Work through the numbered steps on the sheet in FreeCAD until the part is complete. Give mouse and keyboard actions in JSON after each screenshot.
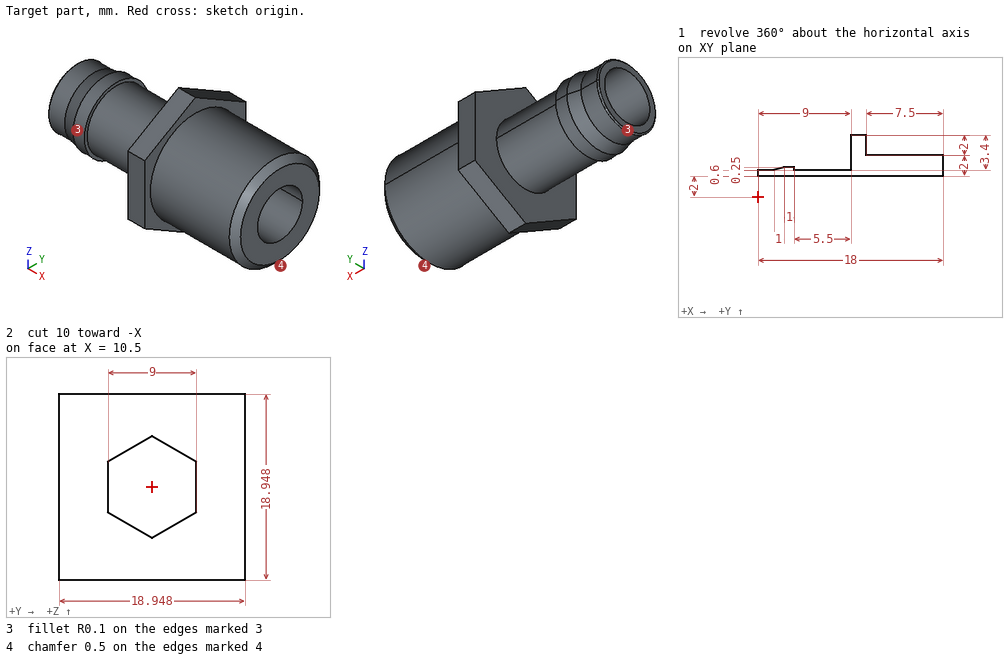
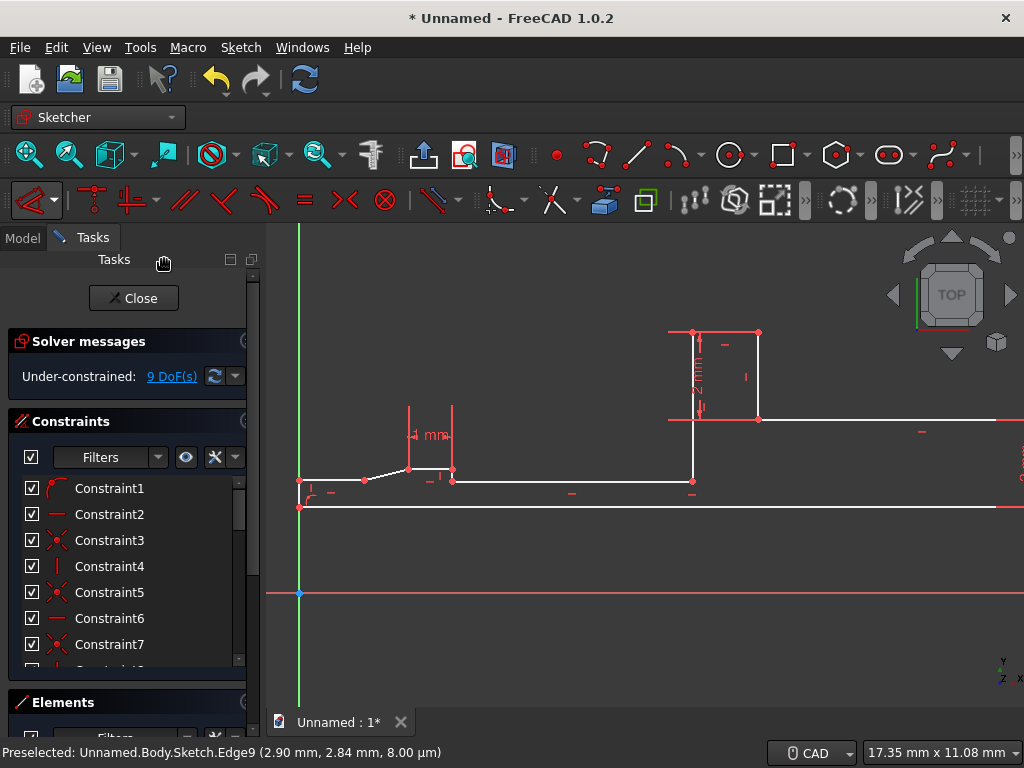
{"action": "left_click", "coordinate": [535, 507]}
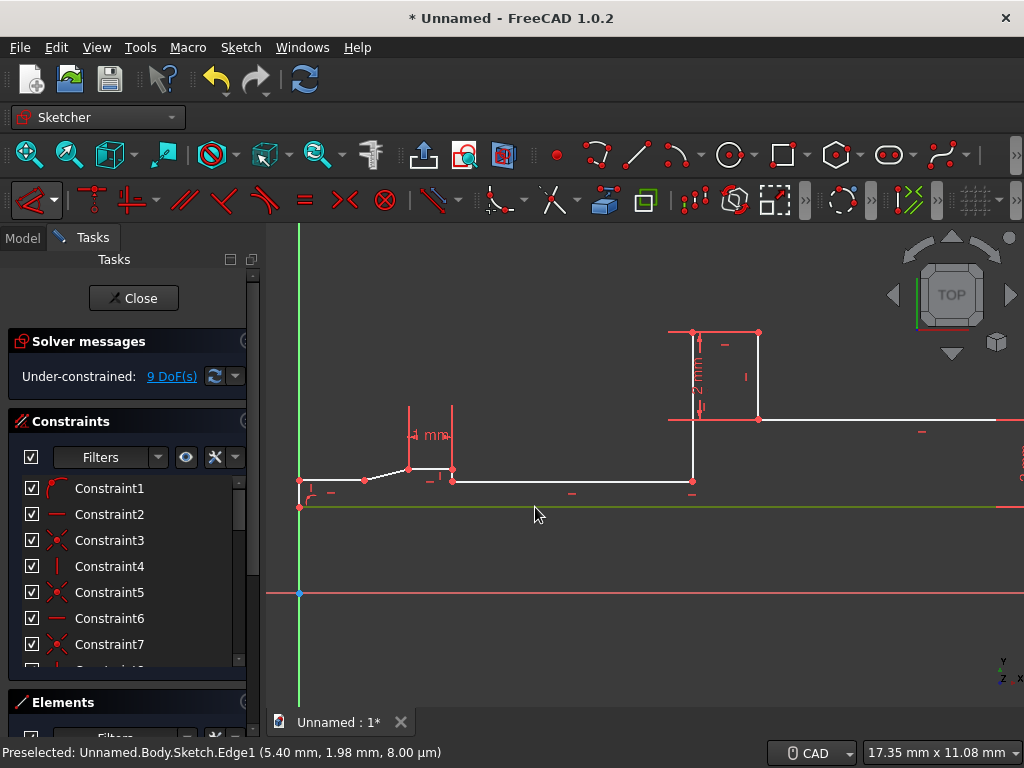
{"action": "key", "text": "l"}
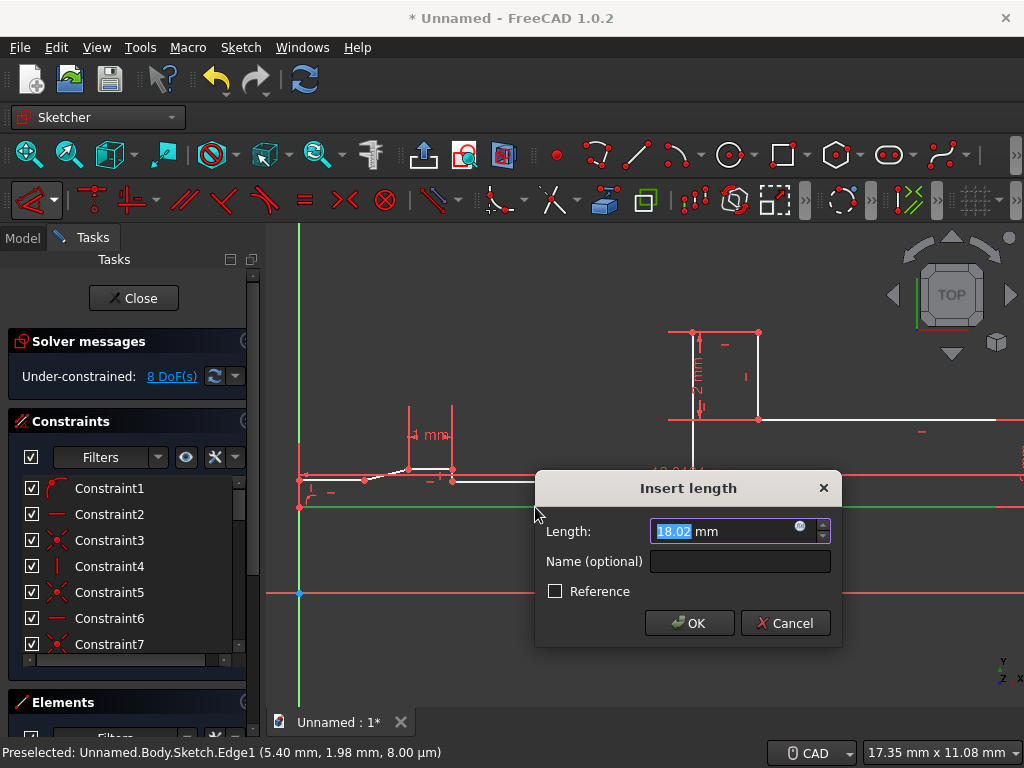
{"action": "type", "text": "18"}
{"action": "key", "text": "Return"}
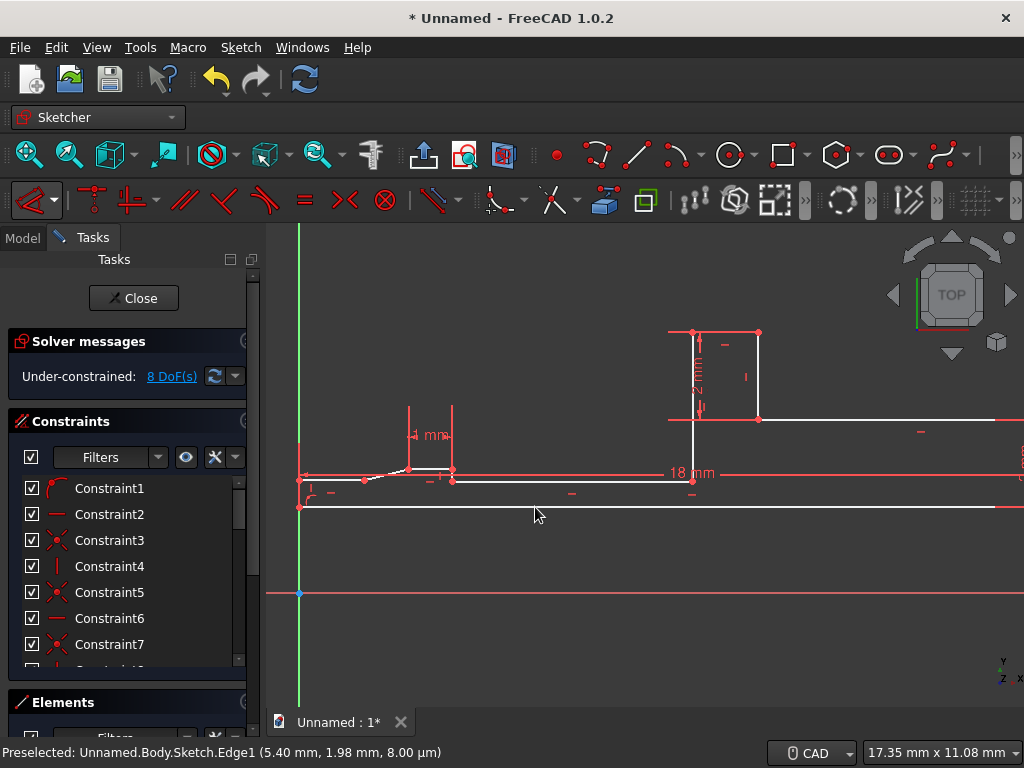
{"action": "left_click", "coordinate": [299, 507]}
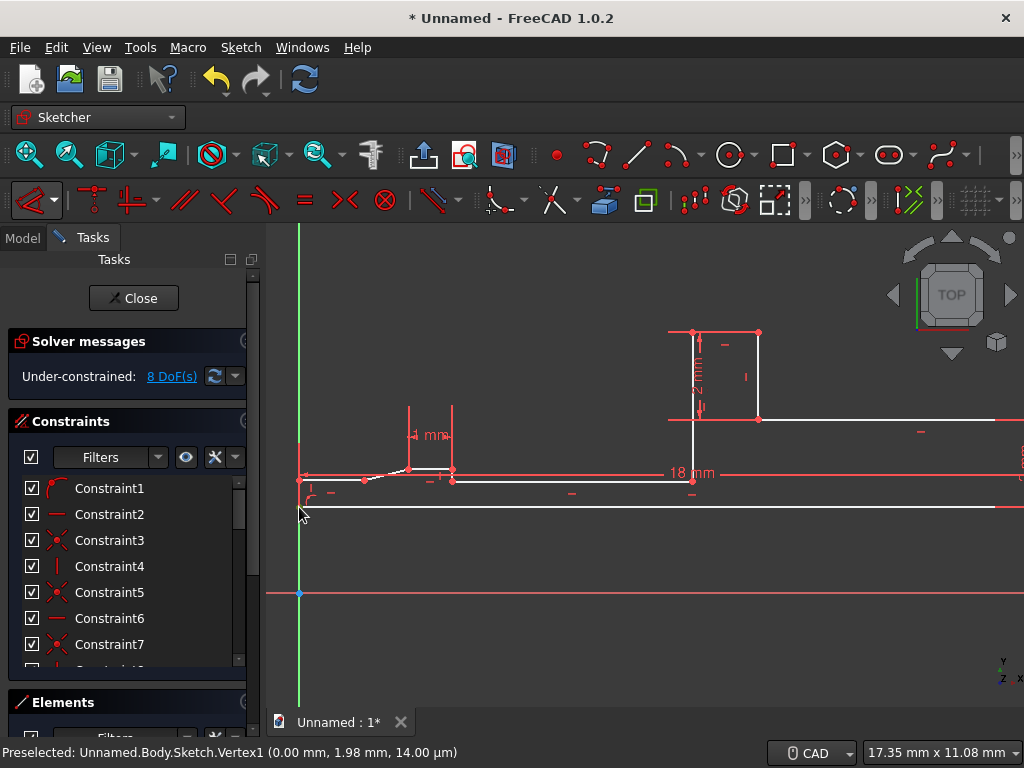
{"action": "left_click", "coordinate": [56, 200]}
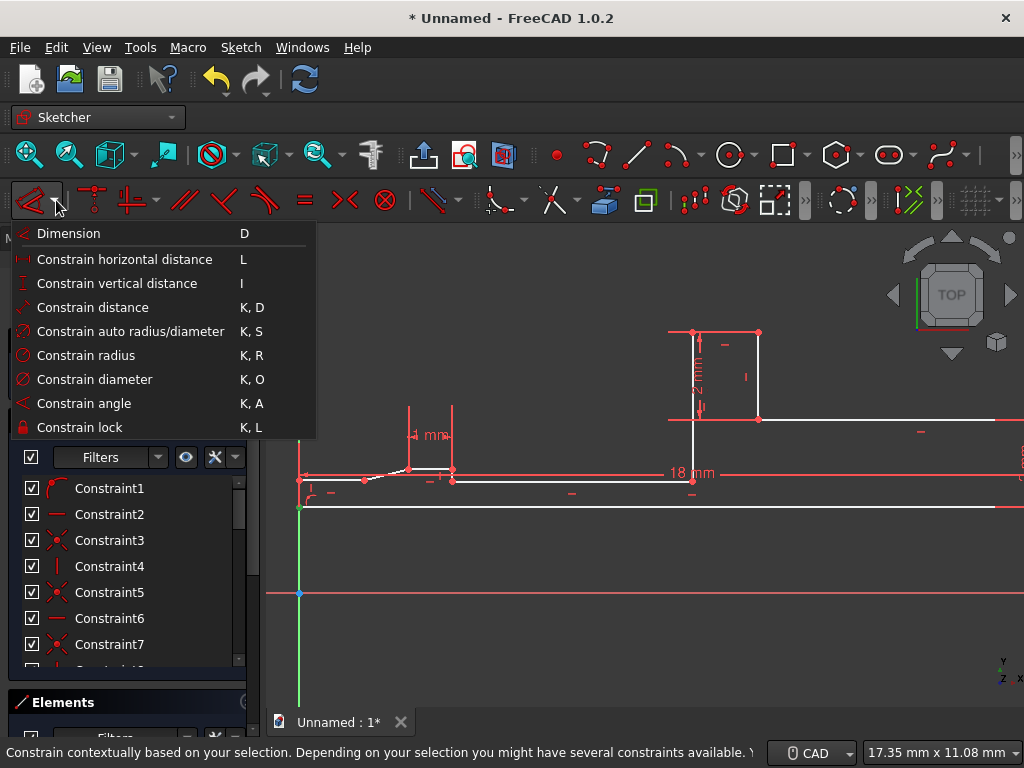
{"action": "left_click", "coordinate": [164, 283]}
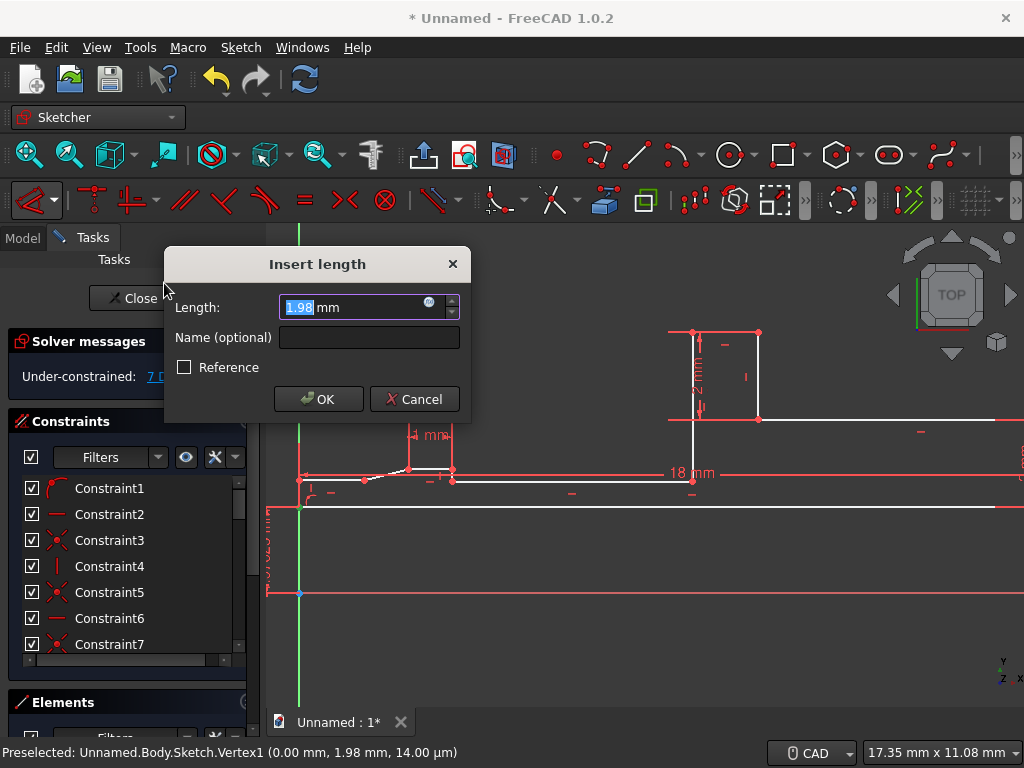
{"action": "type", "text": "2"}
{"action": "key", "text": "Return"}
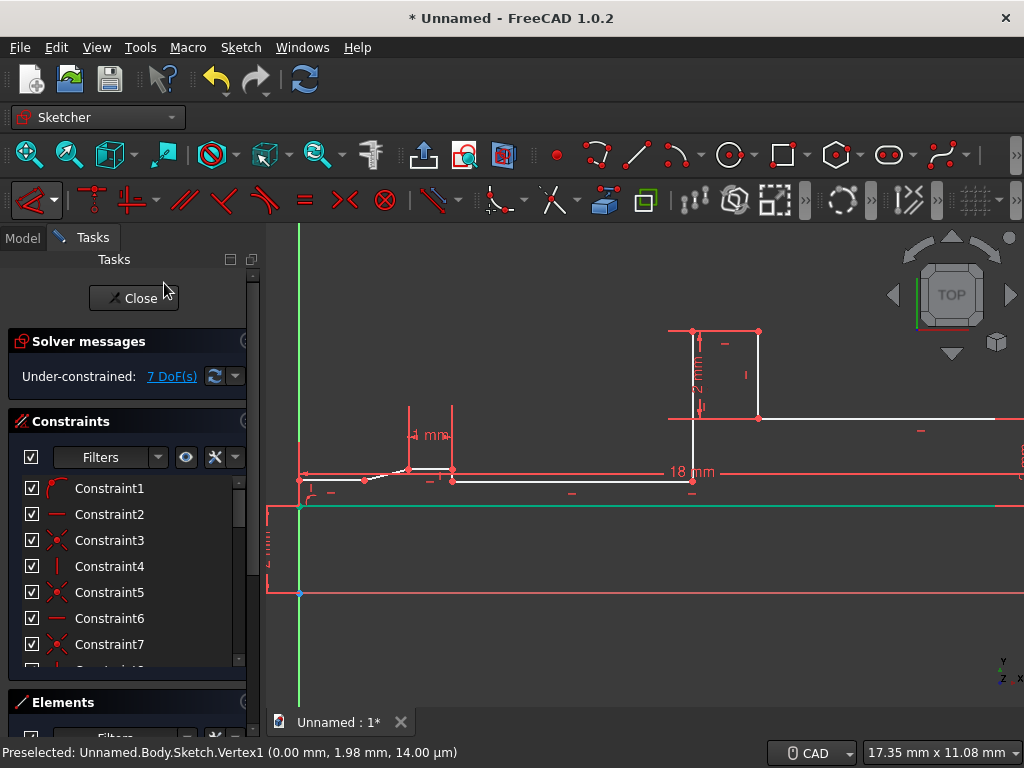
{"action": "left_click", "coordinate": [693, 331]}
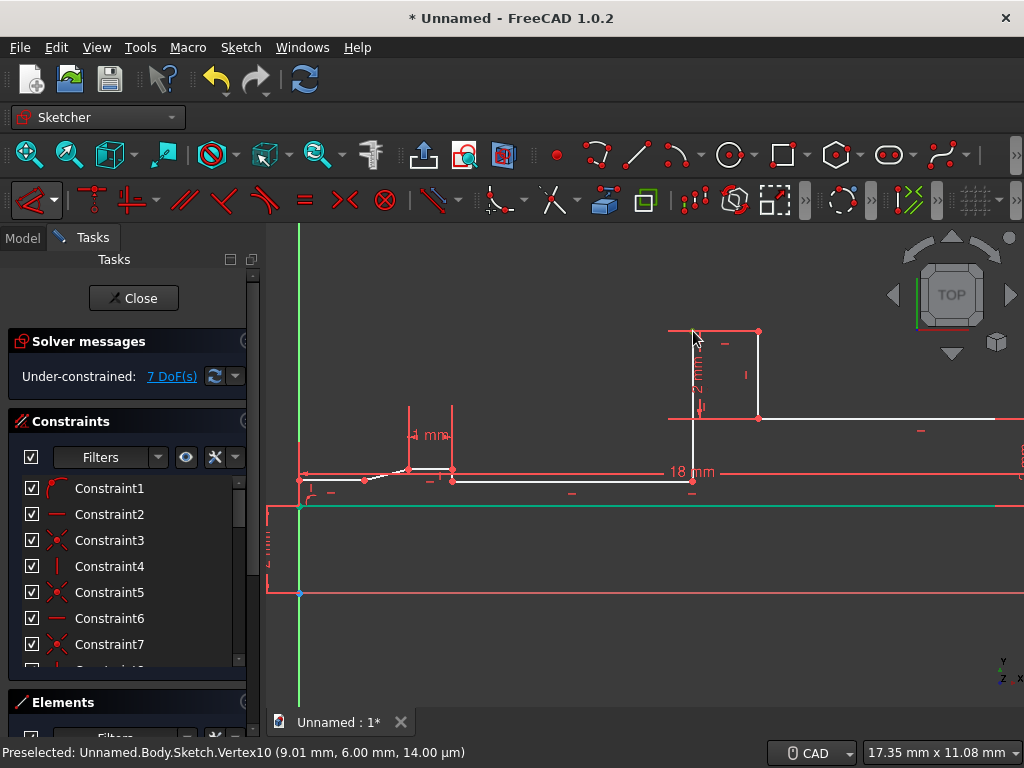
{"action": "left_click", "coordinate": [56, 200]}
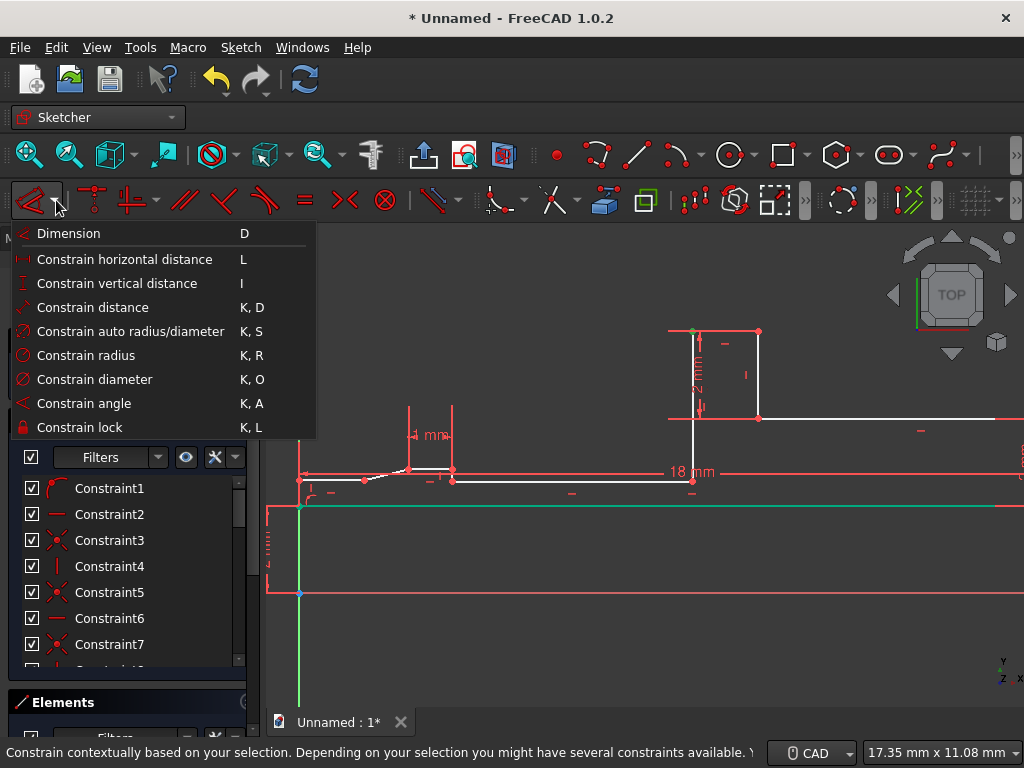
{"action": "left_click", "coordinate": [164, 259]}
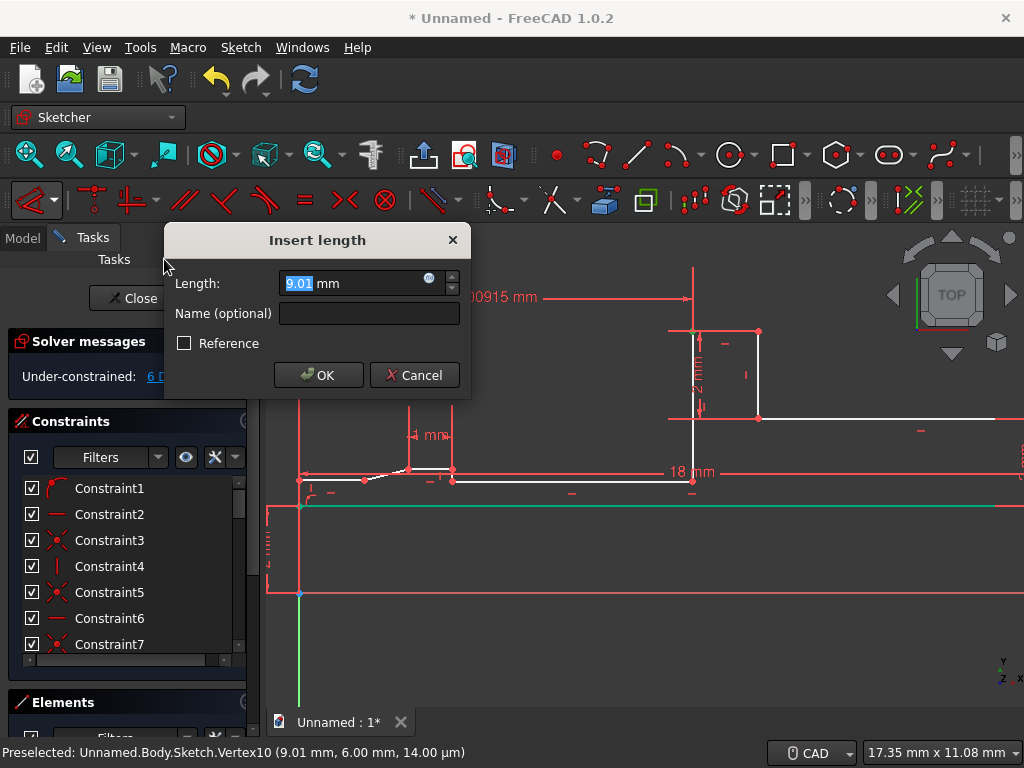
{"action": "type", "text": "9"}
{"action": "key", "text": "Return"}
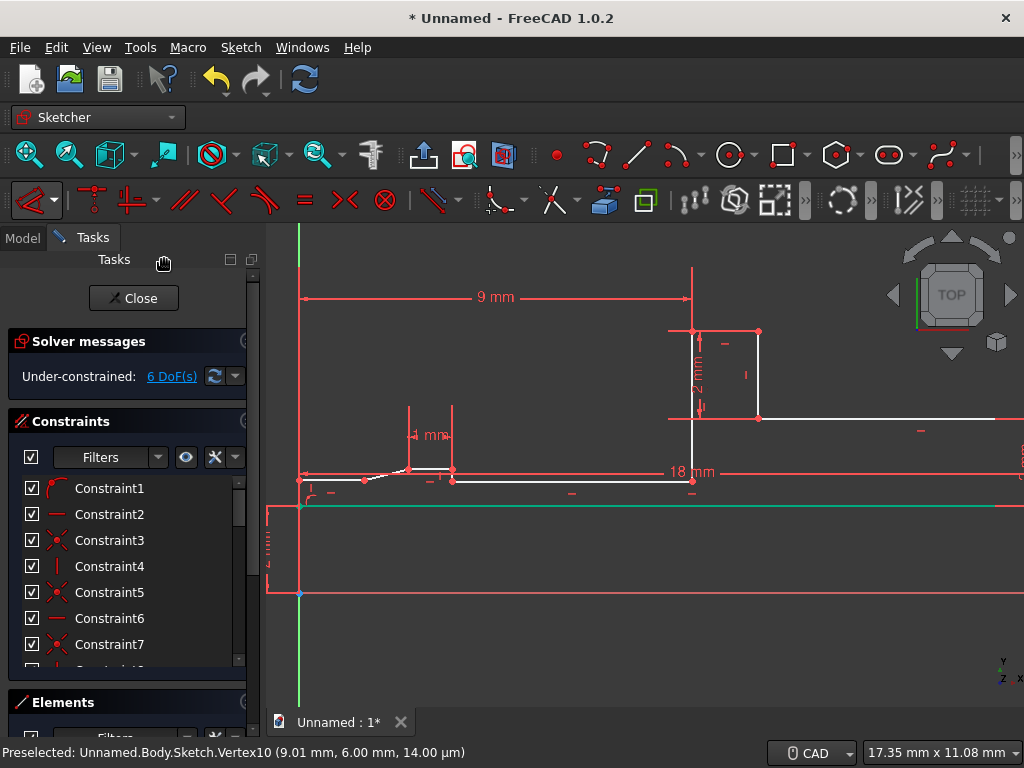
{"action": "left_click", "coordinate": [395, 473]}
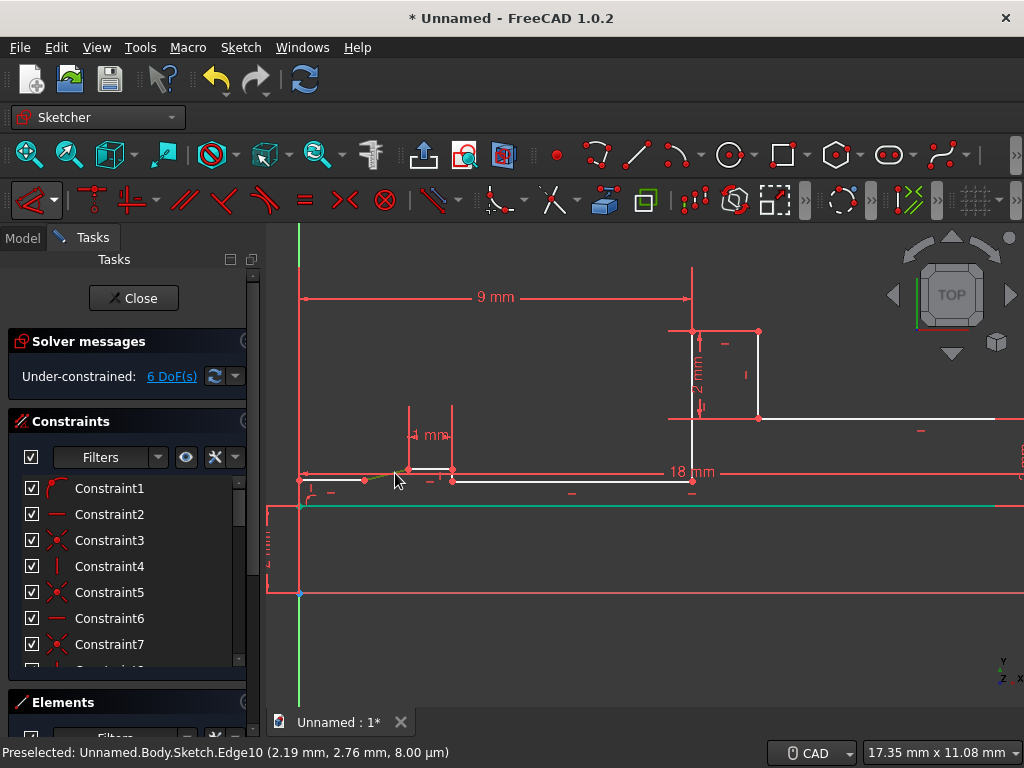
{"action": "key", "text": "l"}